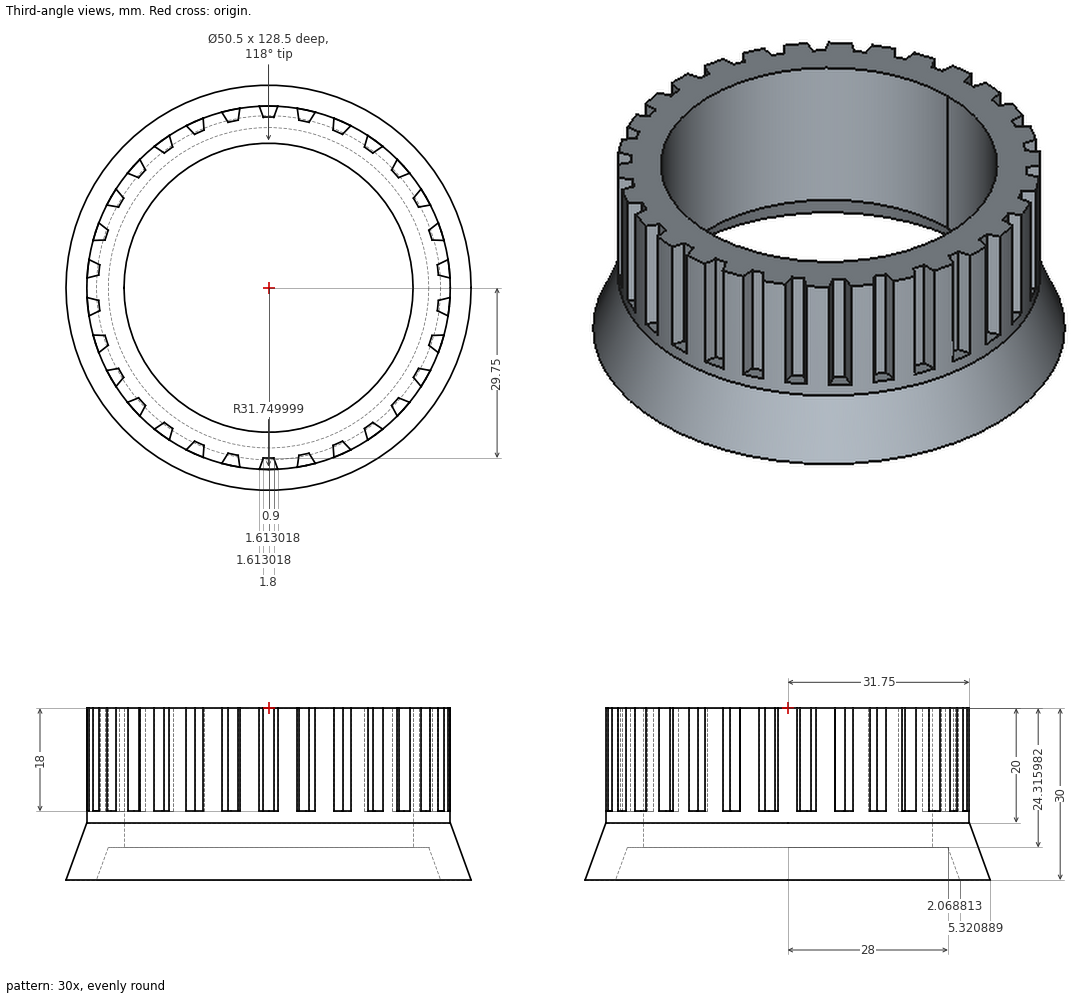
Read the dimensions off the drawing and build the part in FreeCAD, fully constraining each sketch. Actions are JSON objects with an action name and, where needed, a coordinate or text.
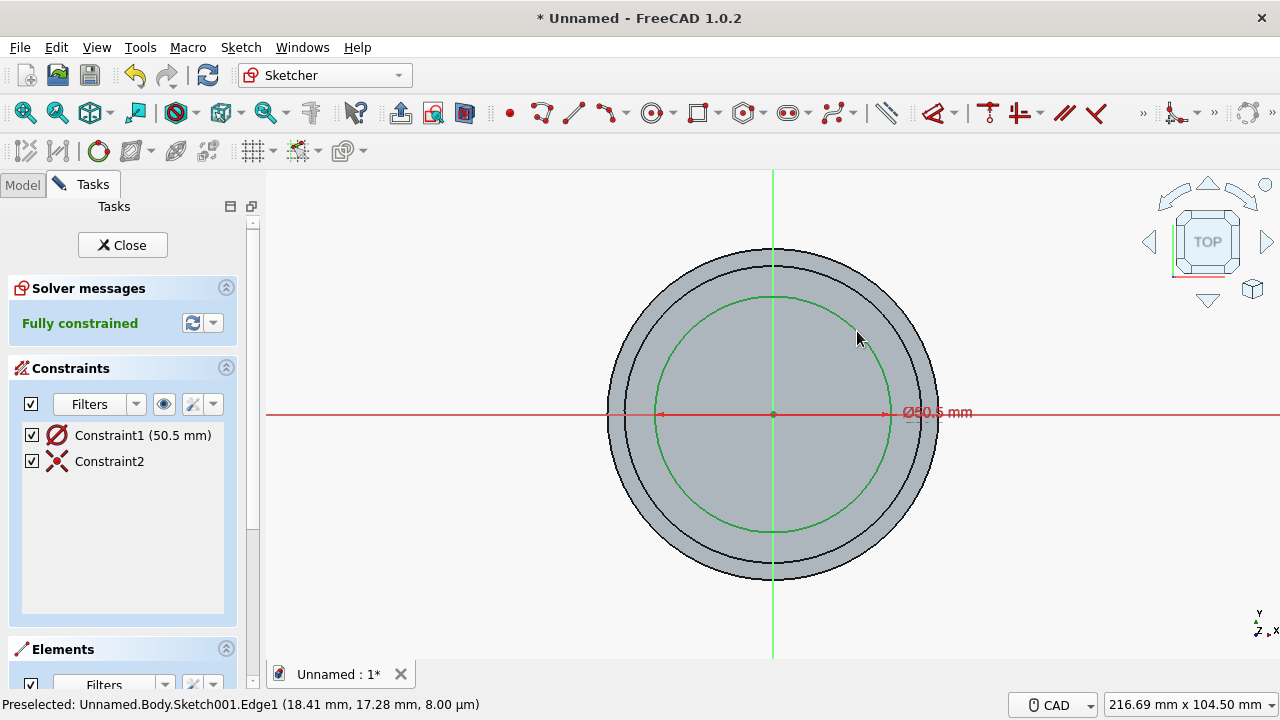
{"action": "left_click", "coordinate": [123, 245]}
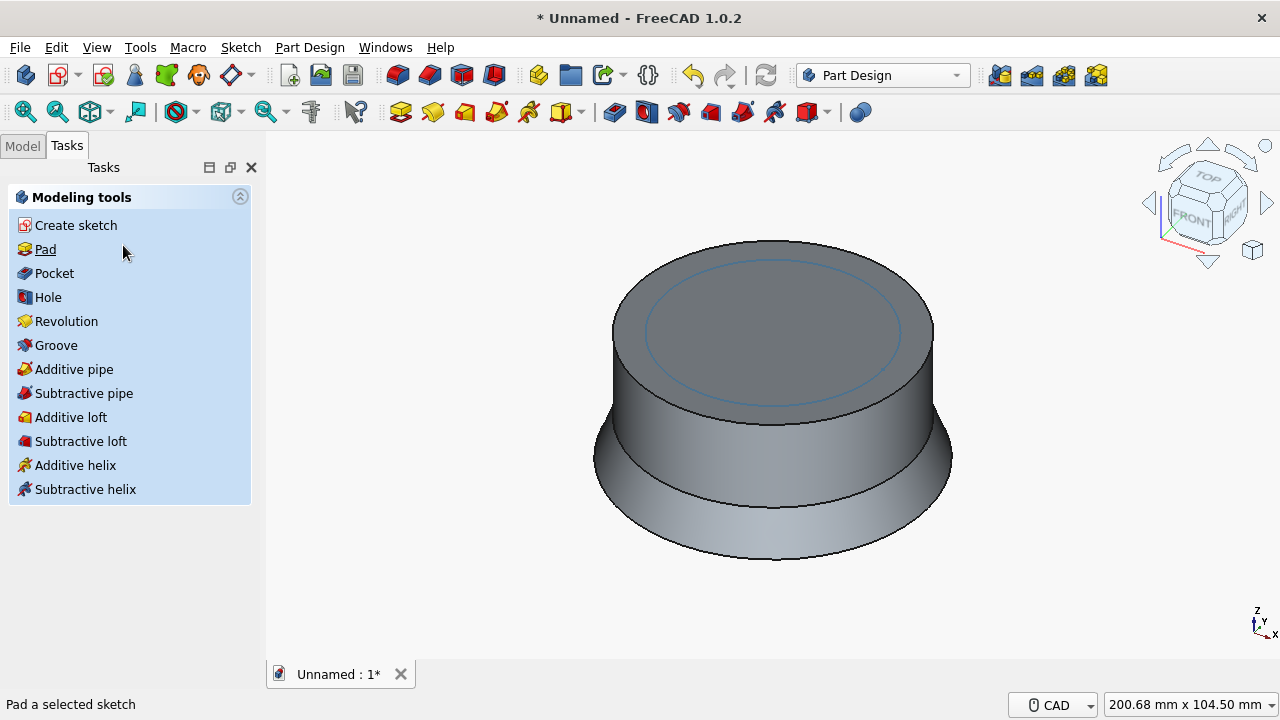
{"action": "left_click", "coordinate": [648, 112]}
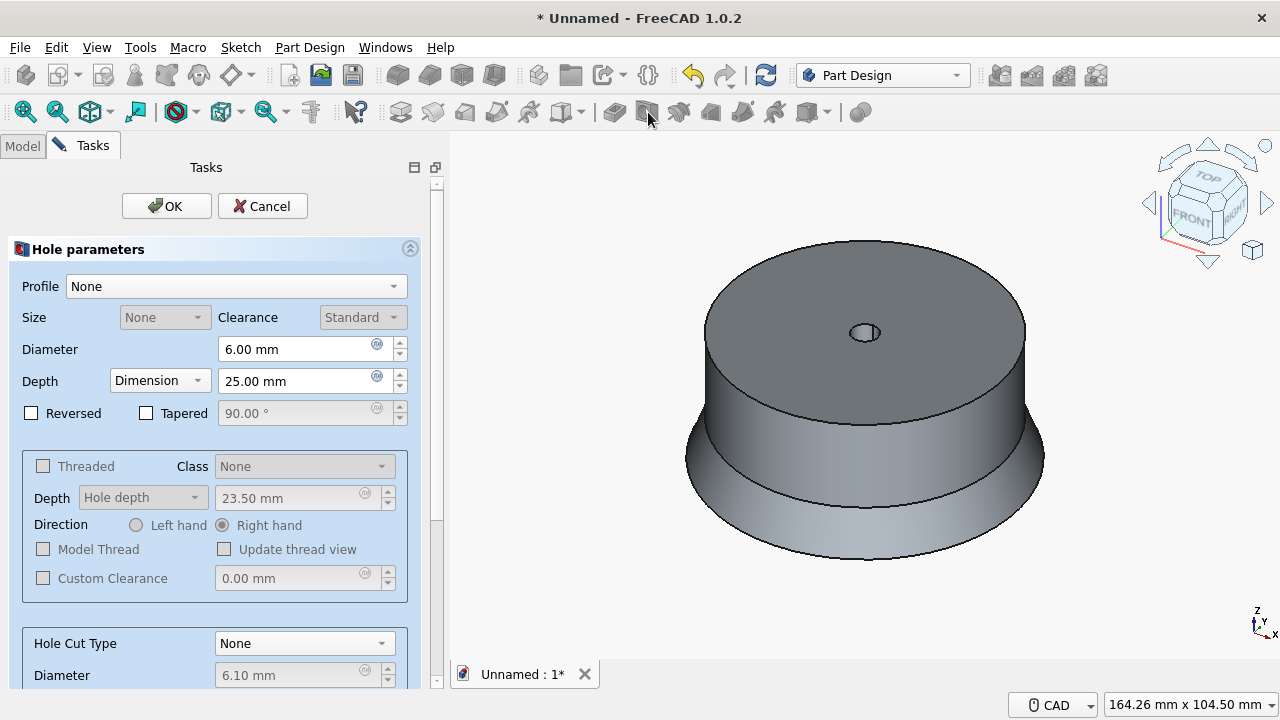
{"action": "triple_click", "coordinate": [305, 349]}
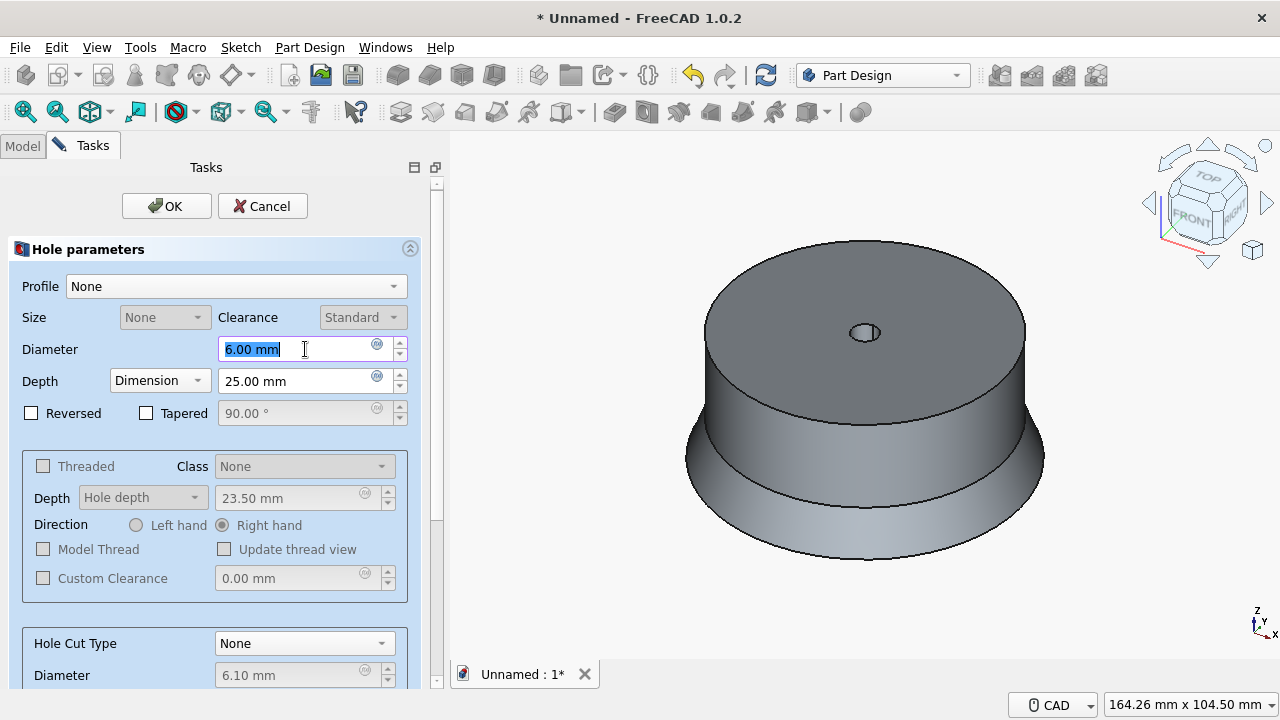
{"action": "type", "text": "50.5"}
{"action": "key", "text": "Tab"}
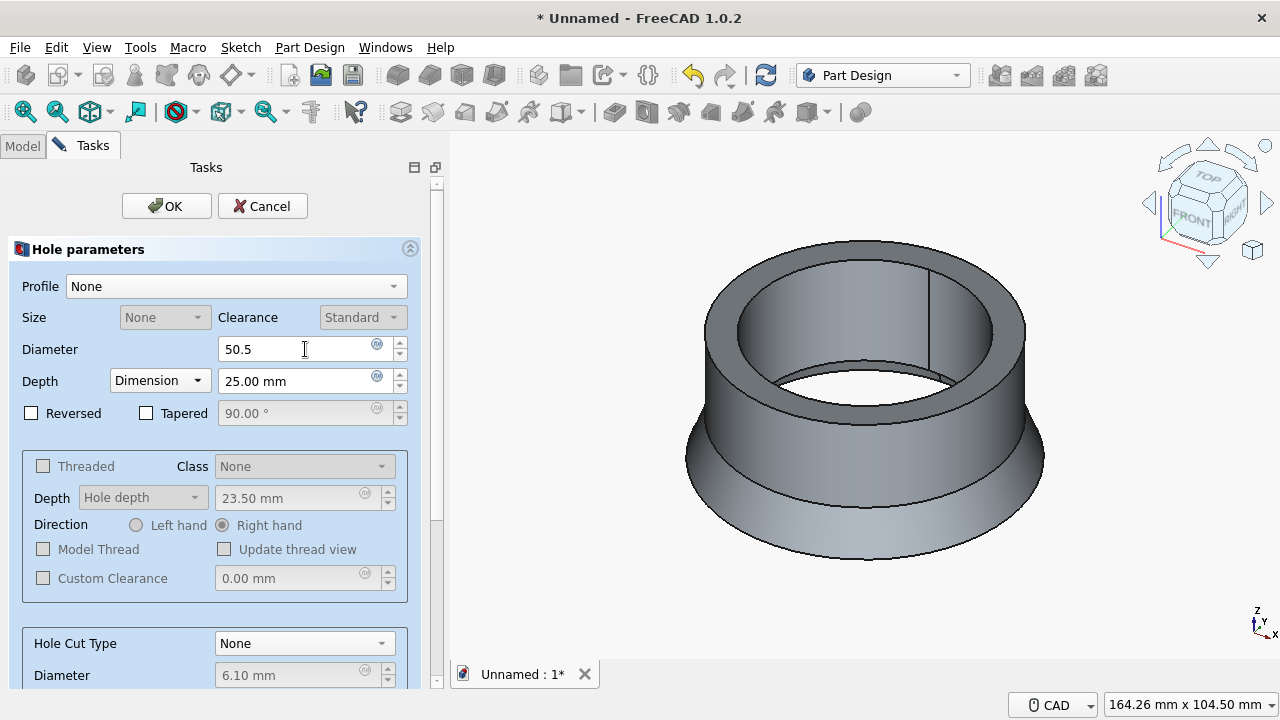
{"action": "triple_click", "coordinate": [305, 381]}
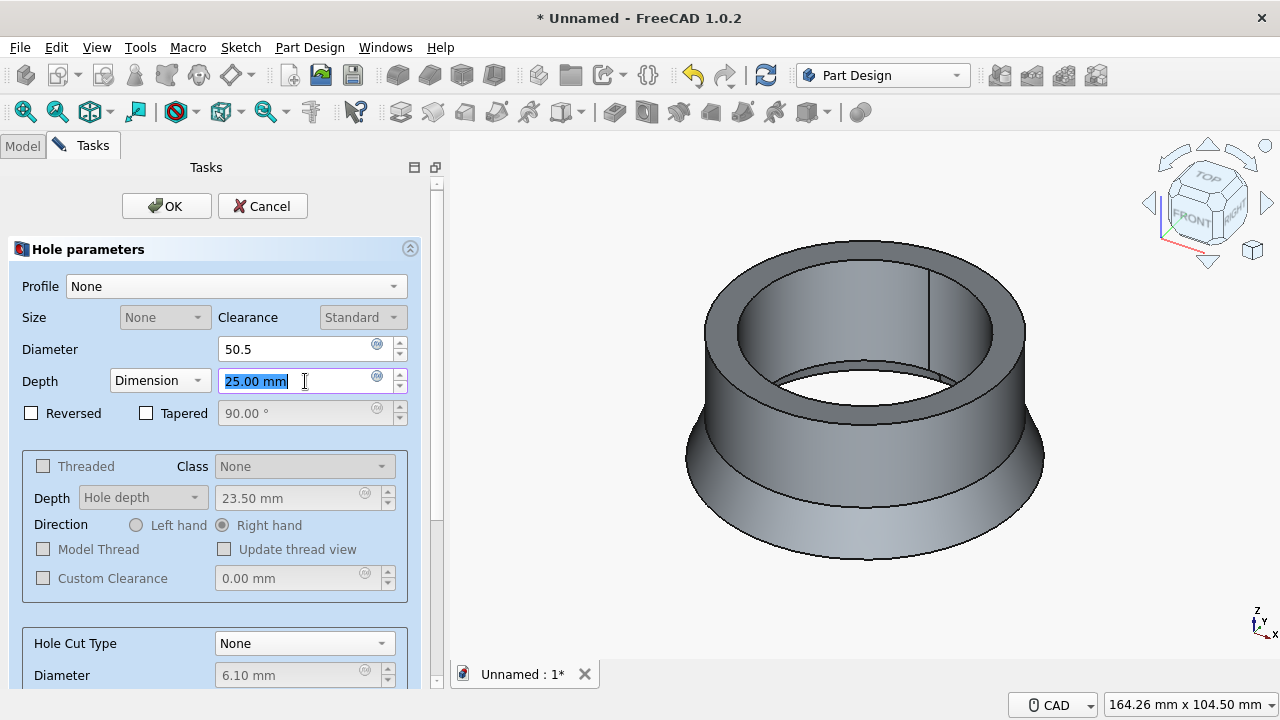
{"action": "type", "text": "128.5"}
{"action": "key", "text": "Tab"}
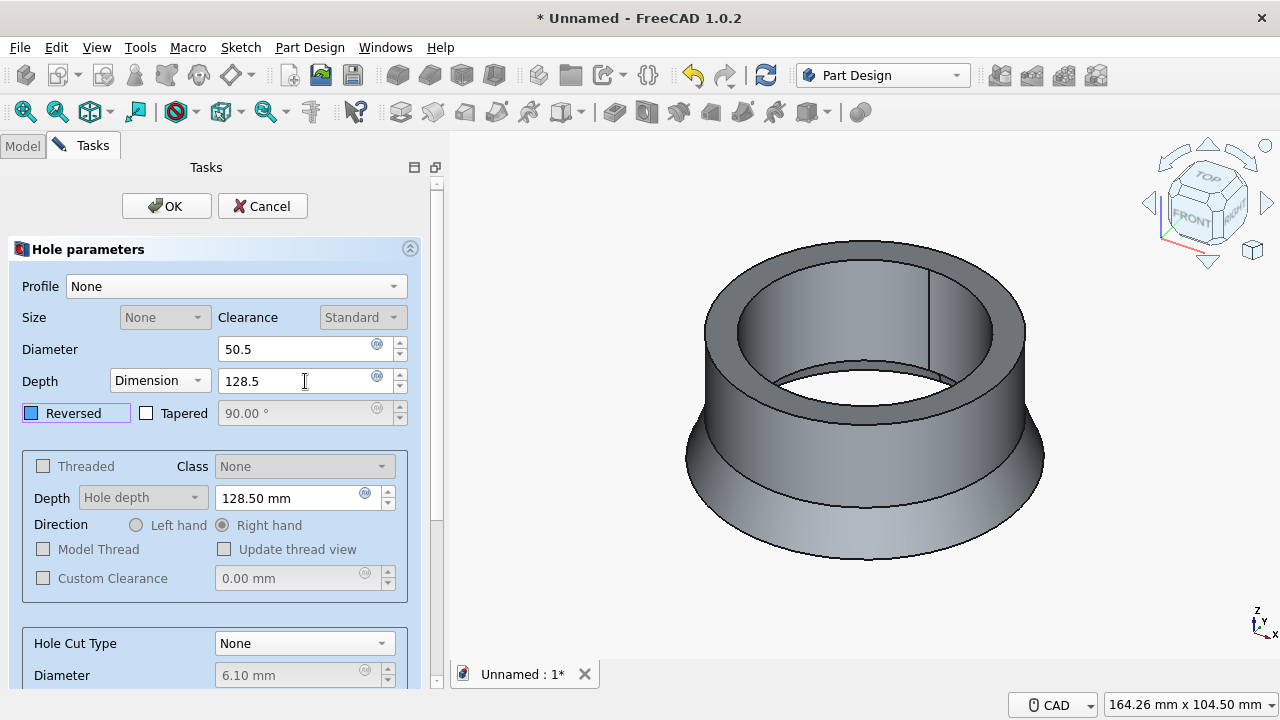
{"action": "left_click", "coordinate": [167, 206]}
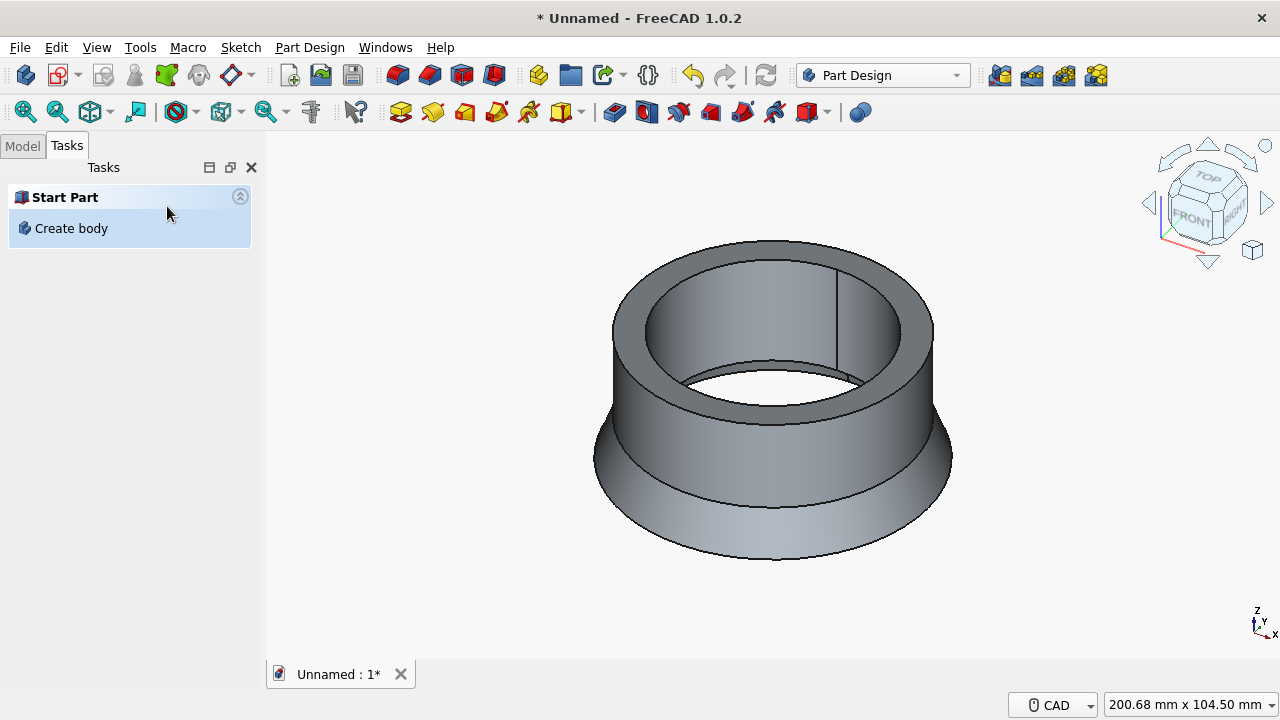
{"action": "left_click", "coordinate": [58, 76]}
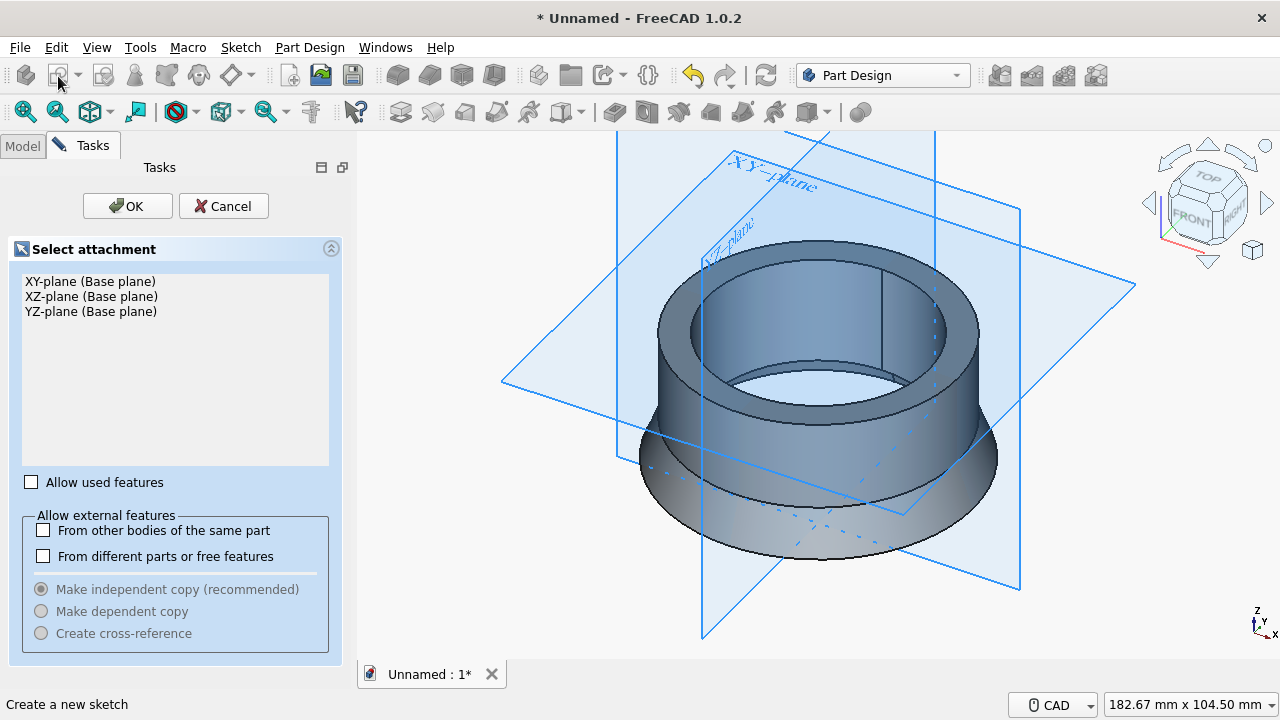
{"action": "left_click", "coordinate": [82, 282]}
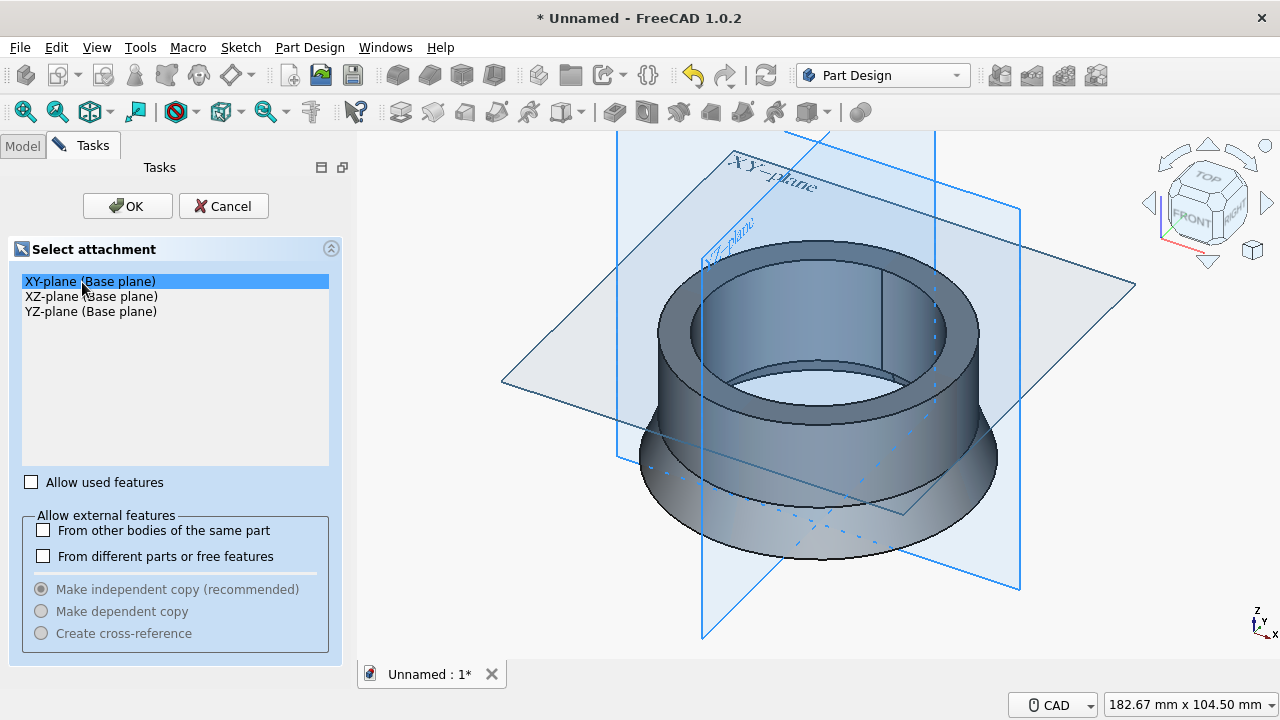
{"action": "left_click", "coordinate": [128, 206]}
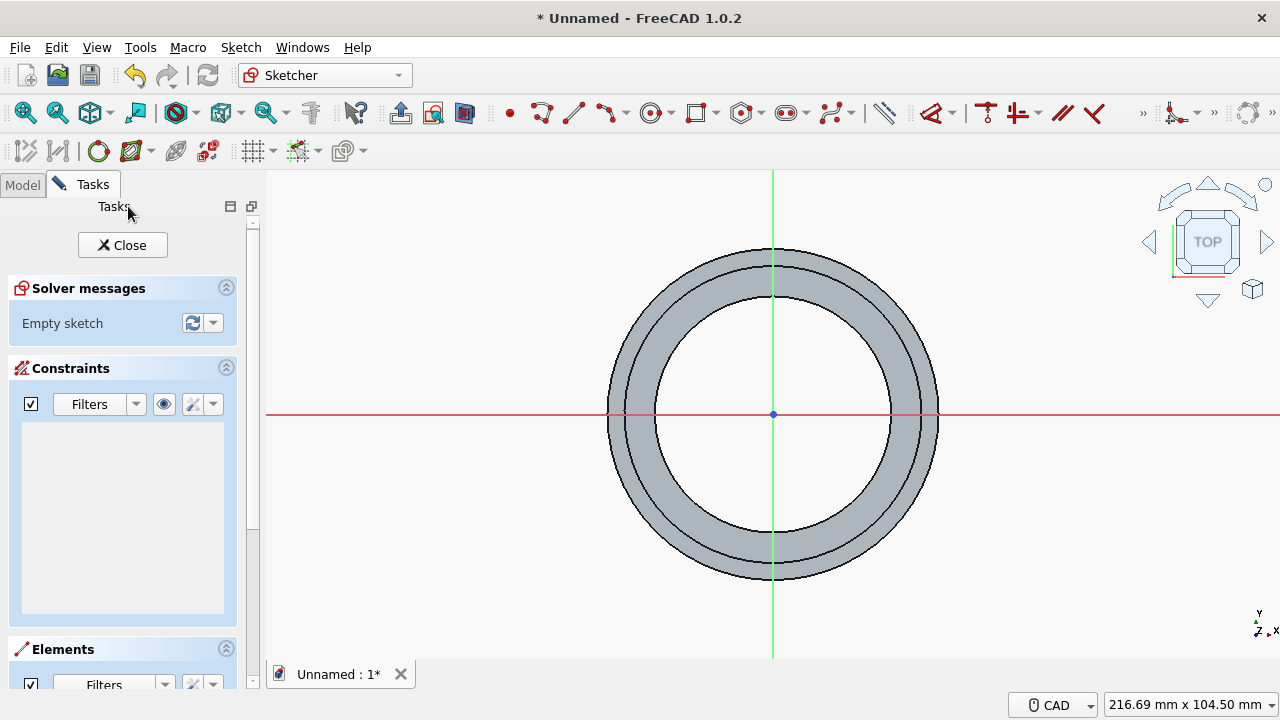
{"action": "scroll", "coordinate": [777, 566], "scroll_direction": "up", "scroll_amount": 15}